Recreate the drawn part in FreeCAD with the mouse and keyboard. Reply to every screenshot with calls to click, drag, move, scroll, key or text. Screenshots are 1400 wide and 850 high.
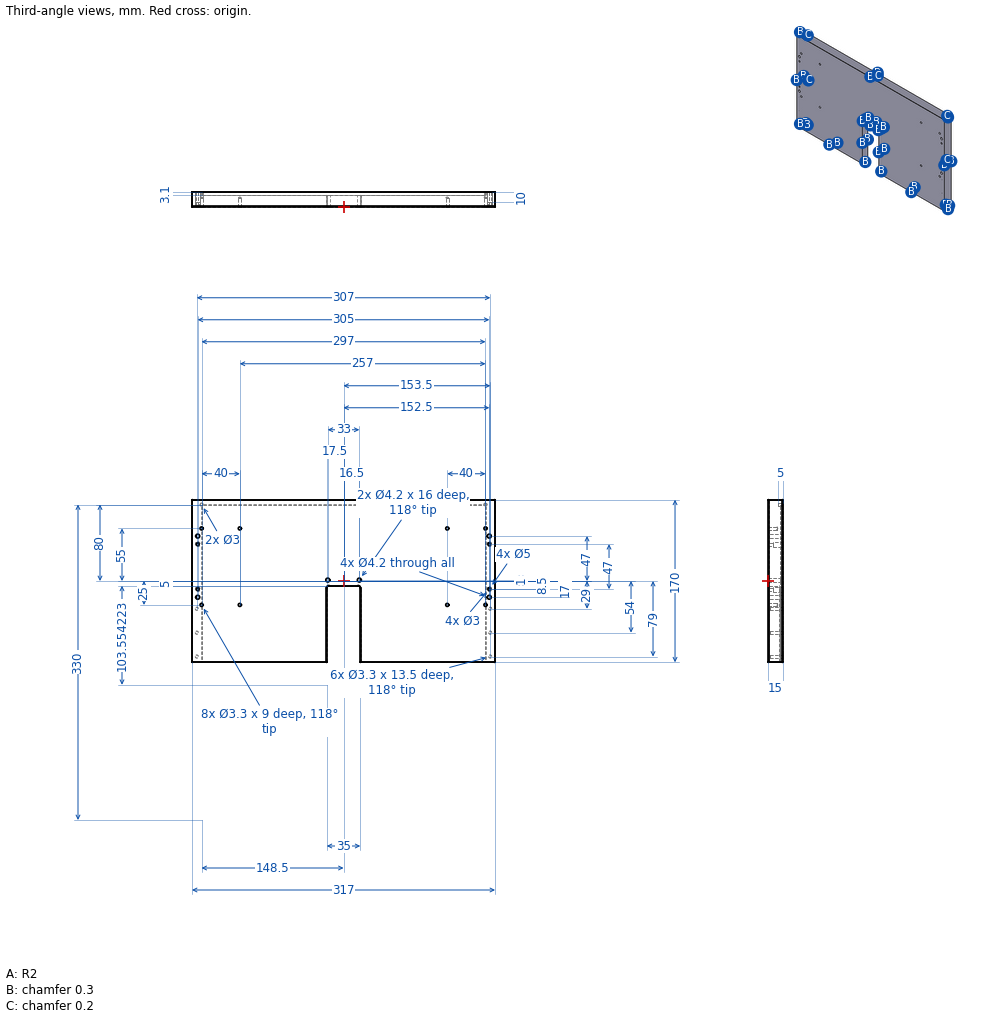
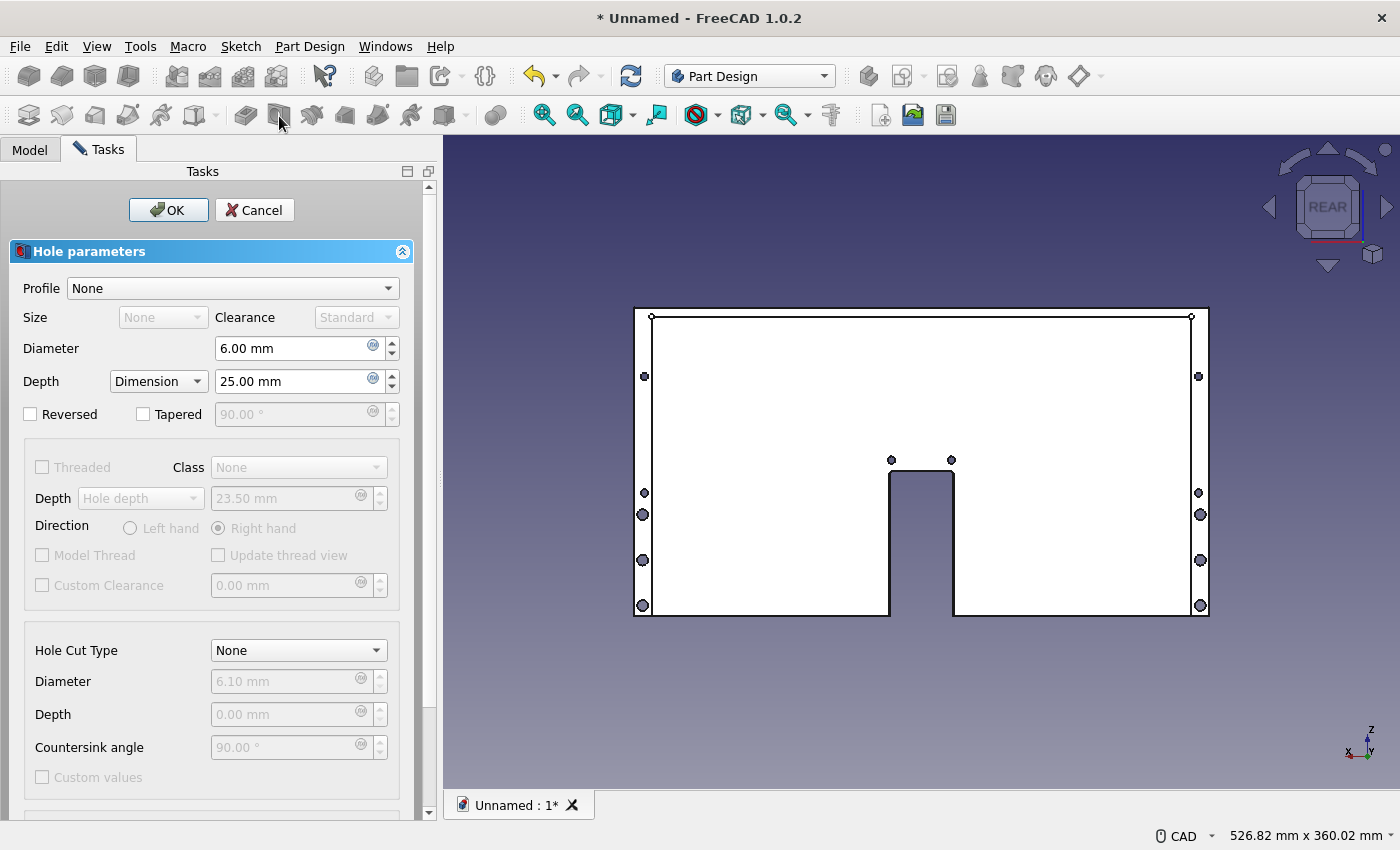
triple_click(300, 348)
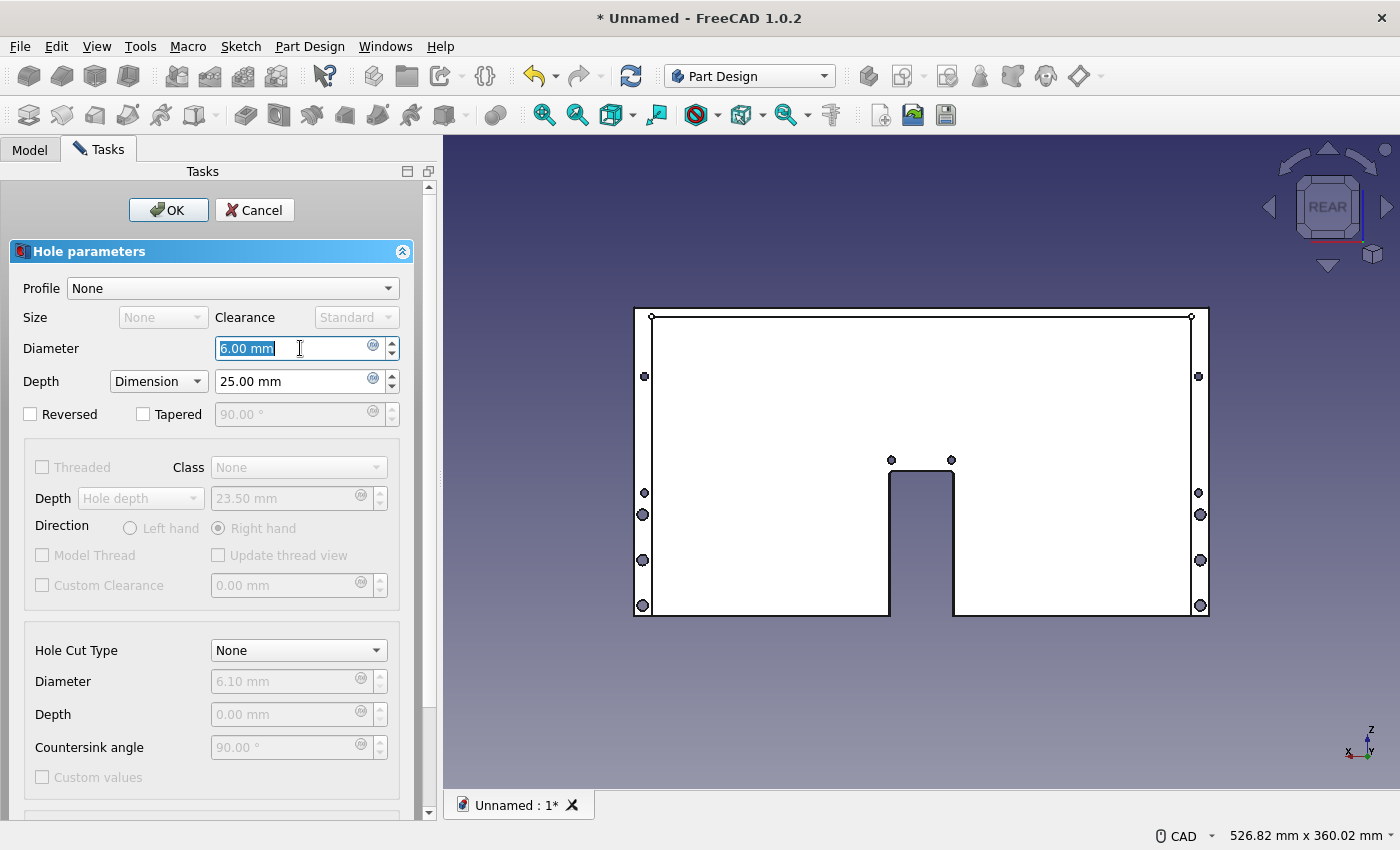
text(3.3)
key(Tab)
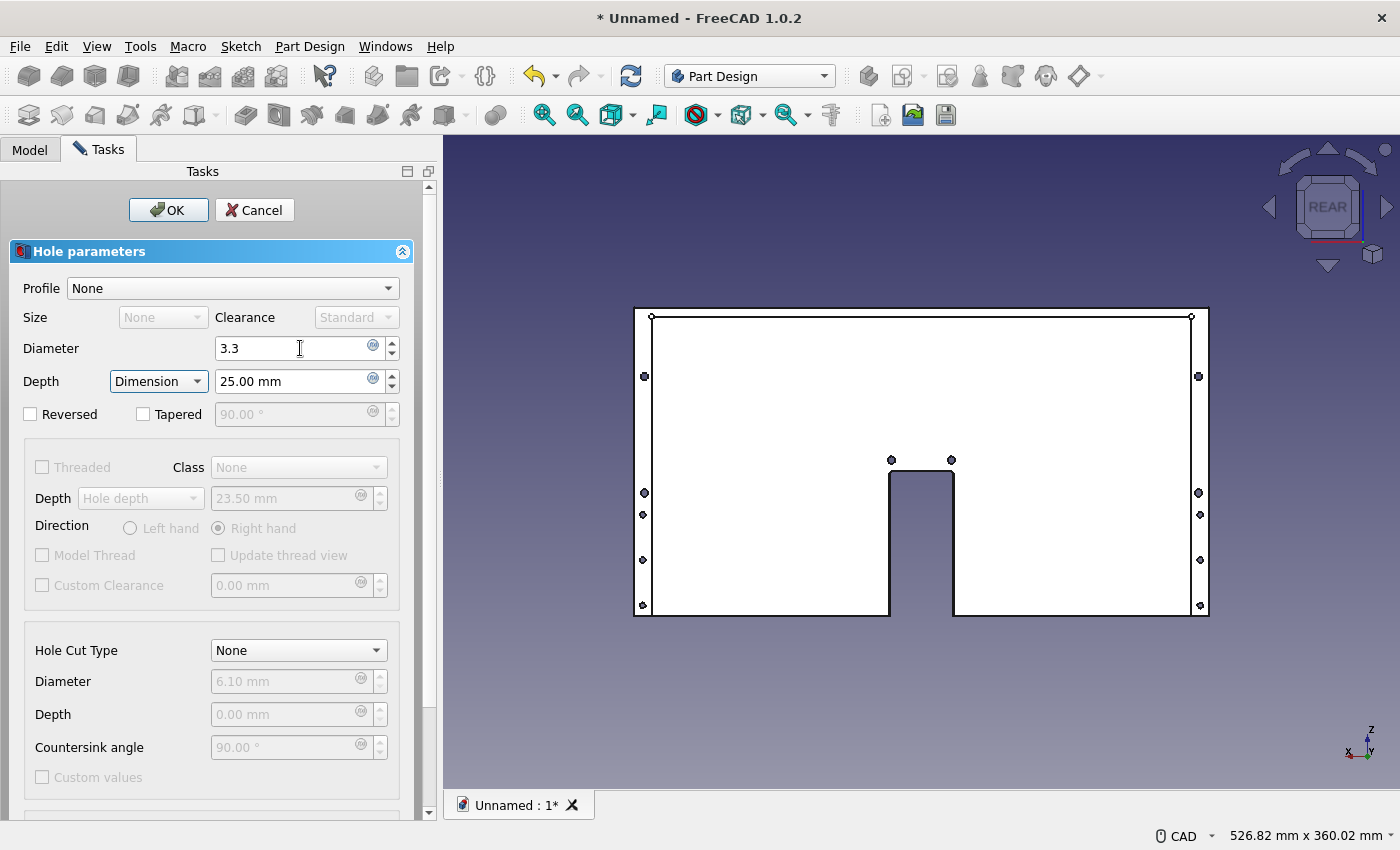
triple_click(300, 382)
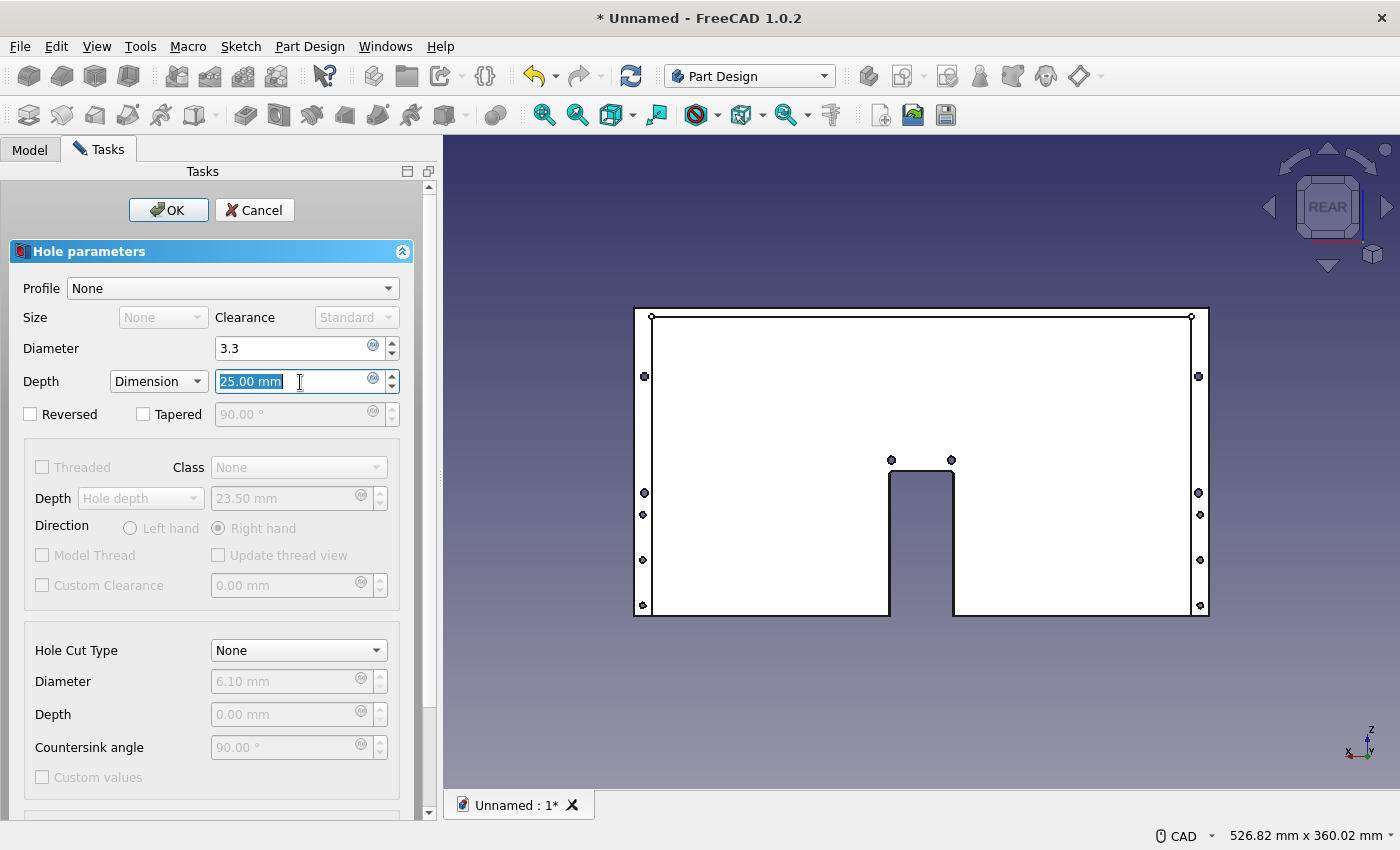
text(13.5)
key(Tab)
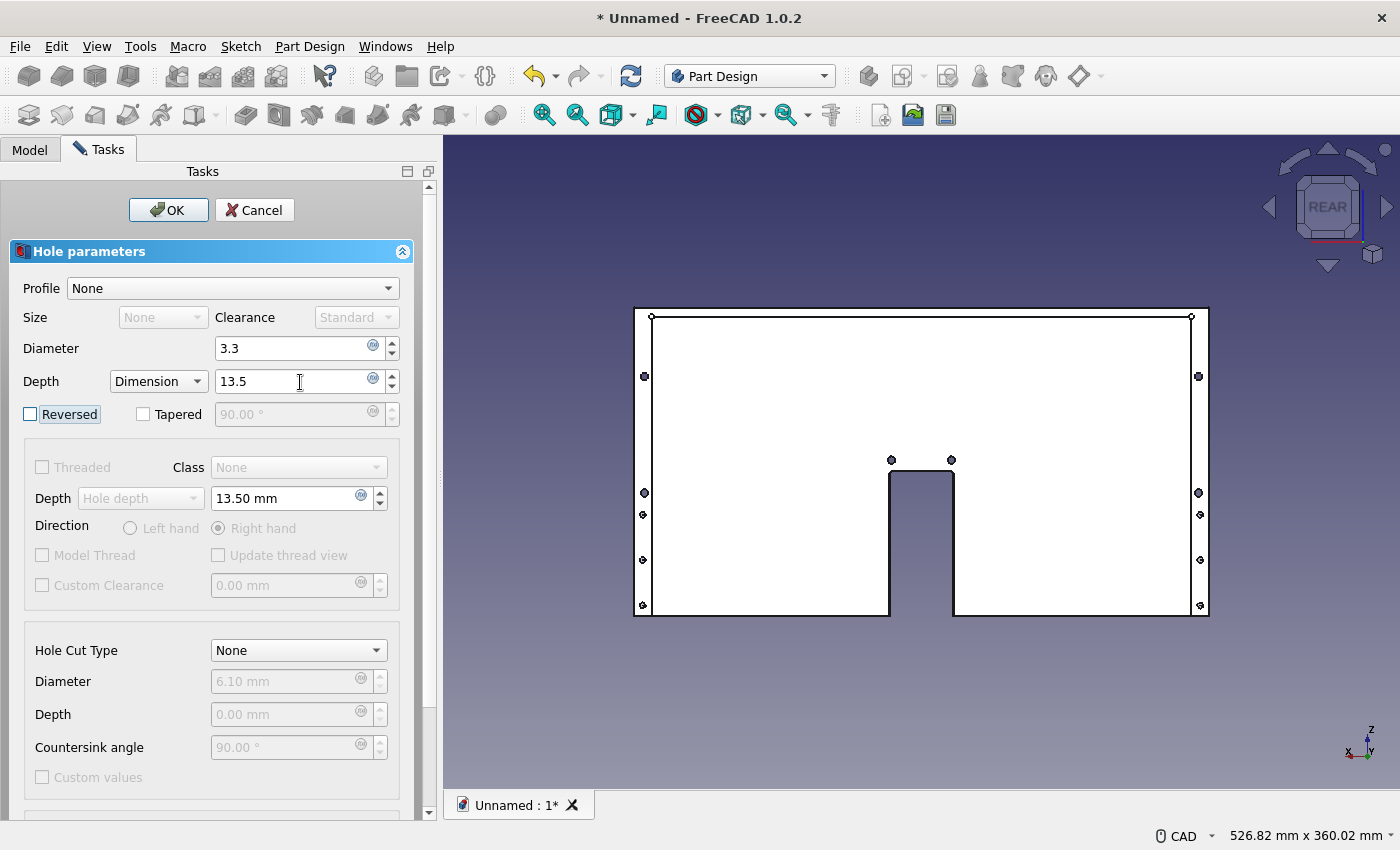
click(169, 210)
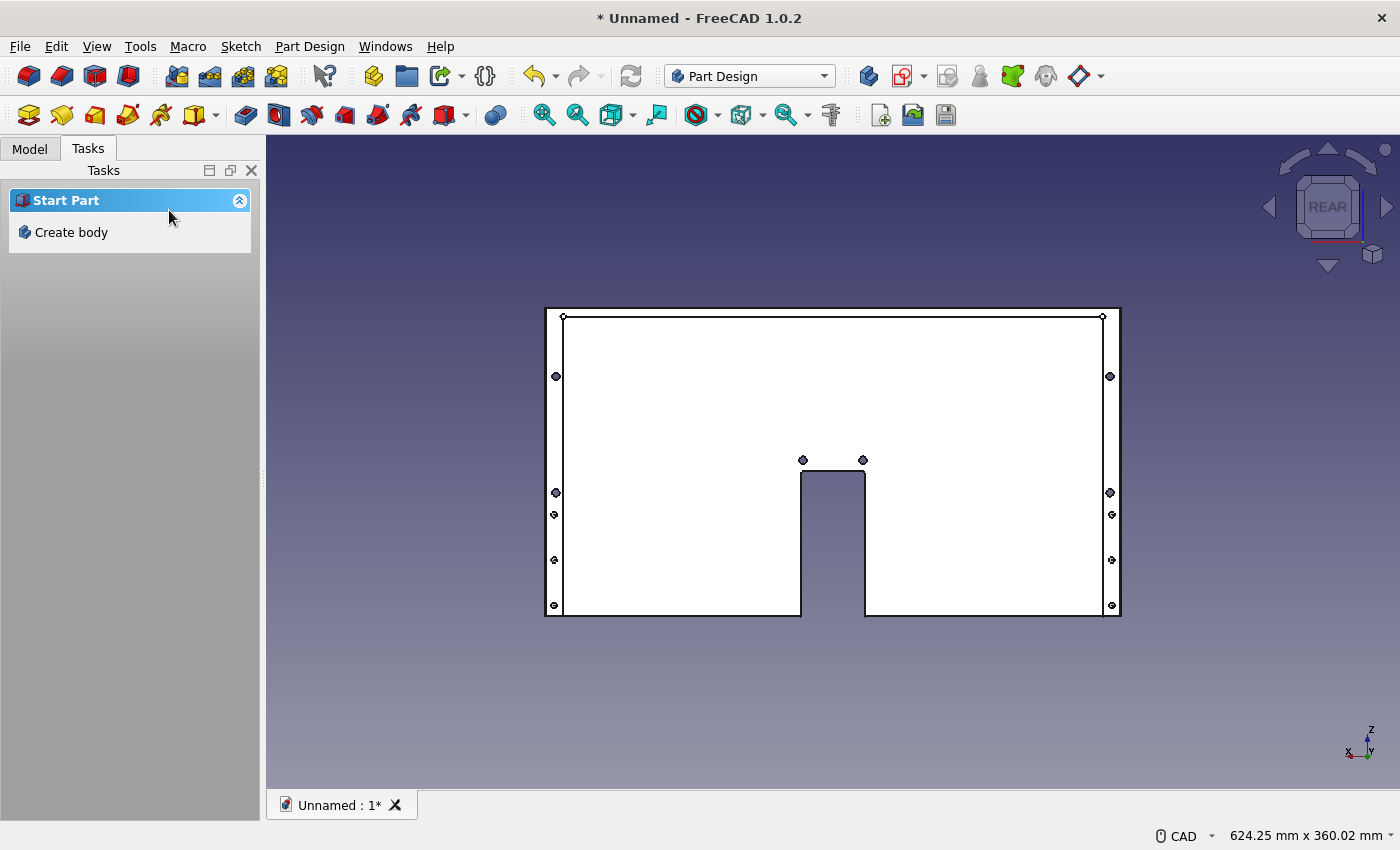
click(1111, 575)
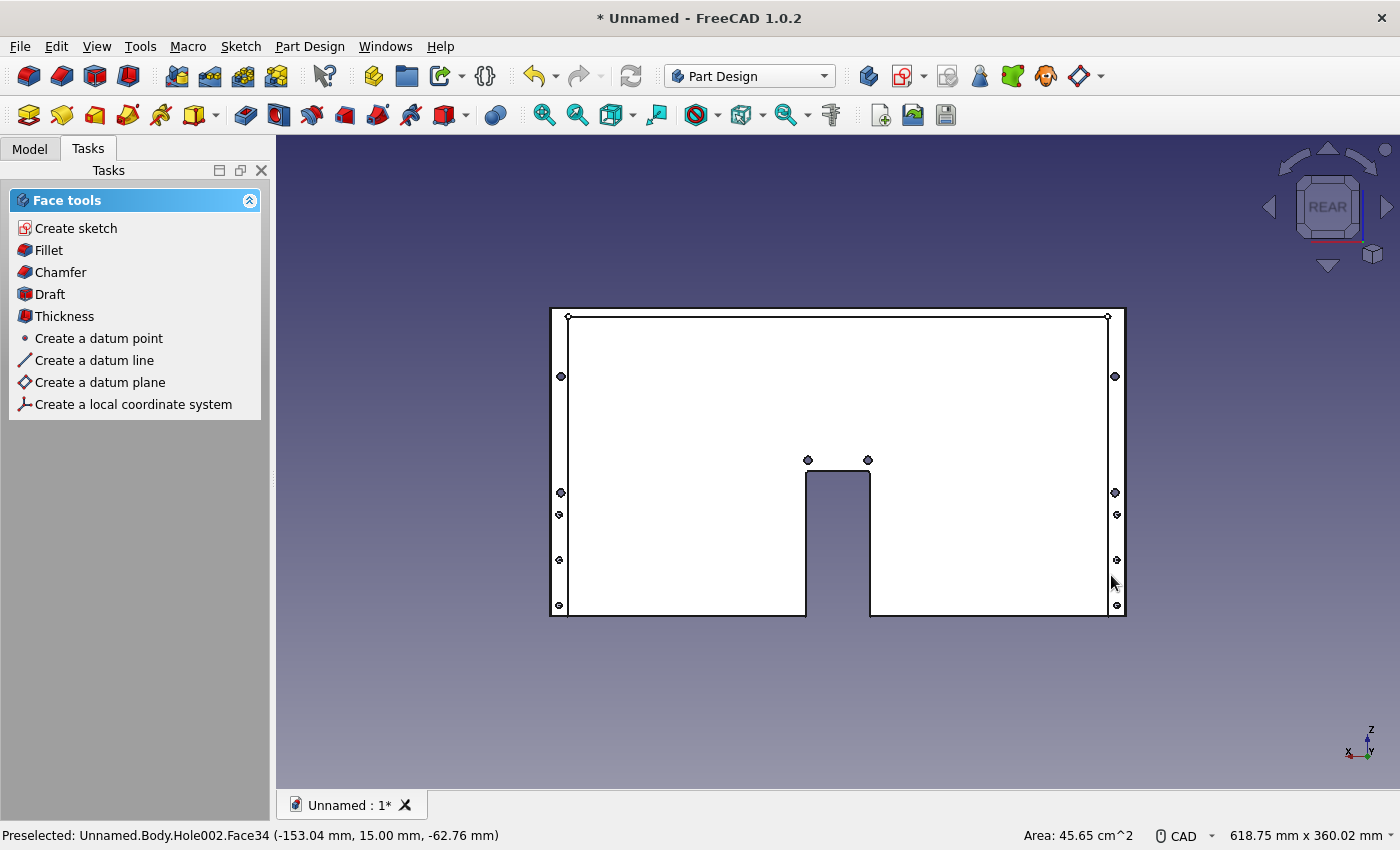
click(902, 76)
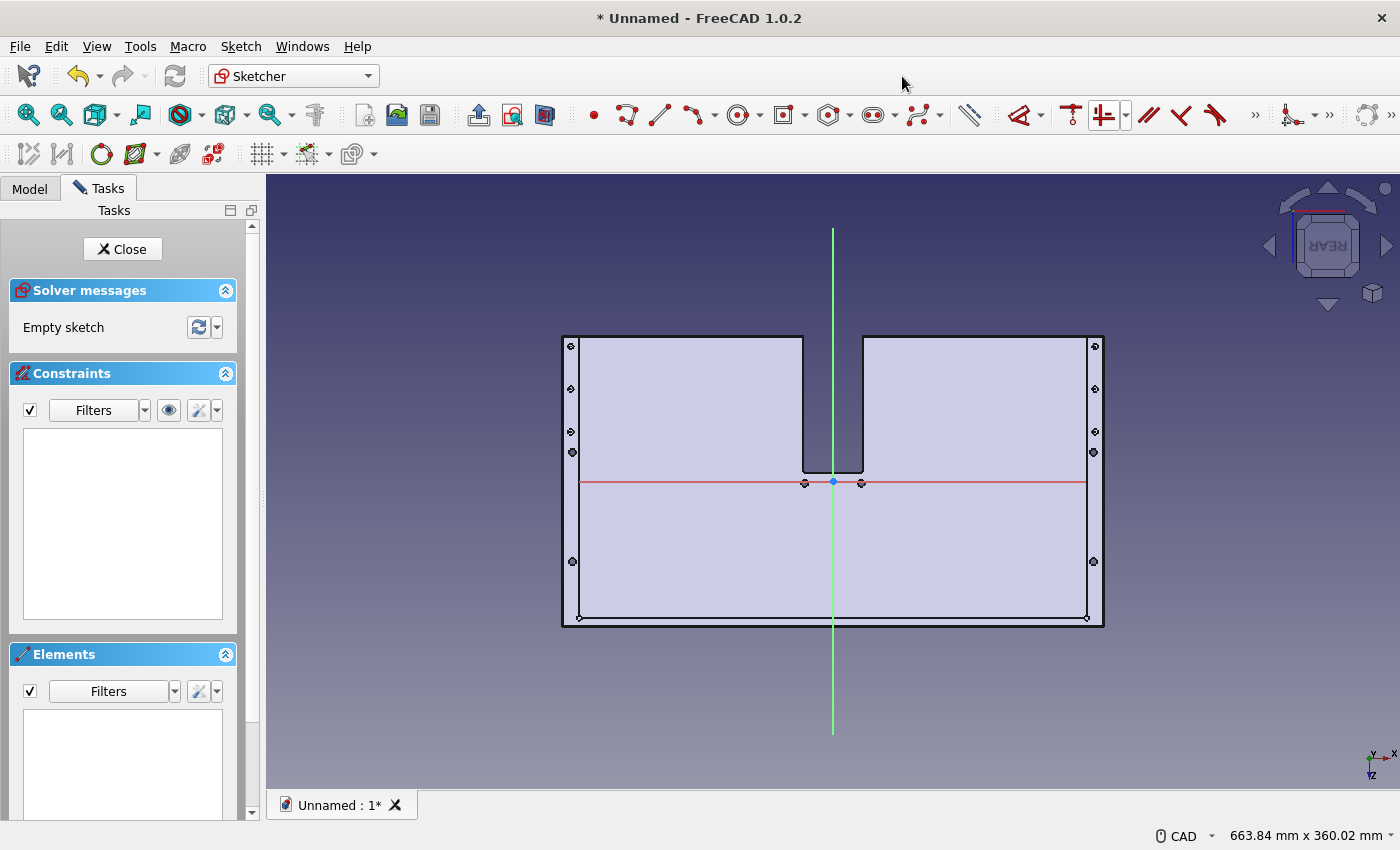
click(738, 116)